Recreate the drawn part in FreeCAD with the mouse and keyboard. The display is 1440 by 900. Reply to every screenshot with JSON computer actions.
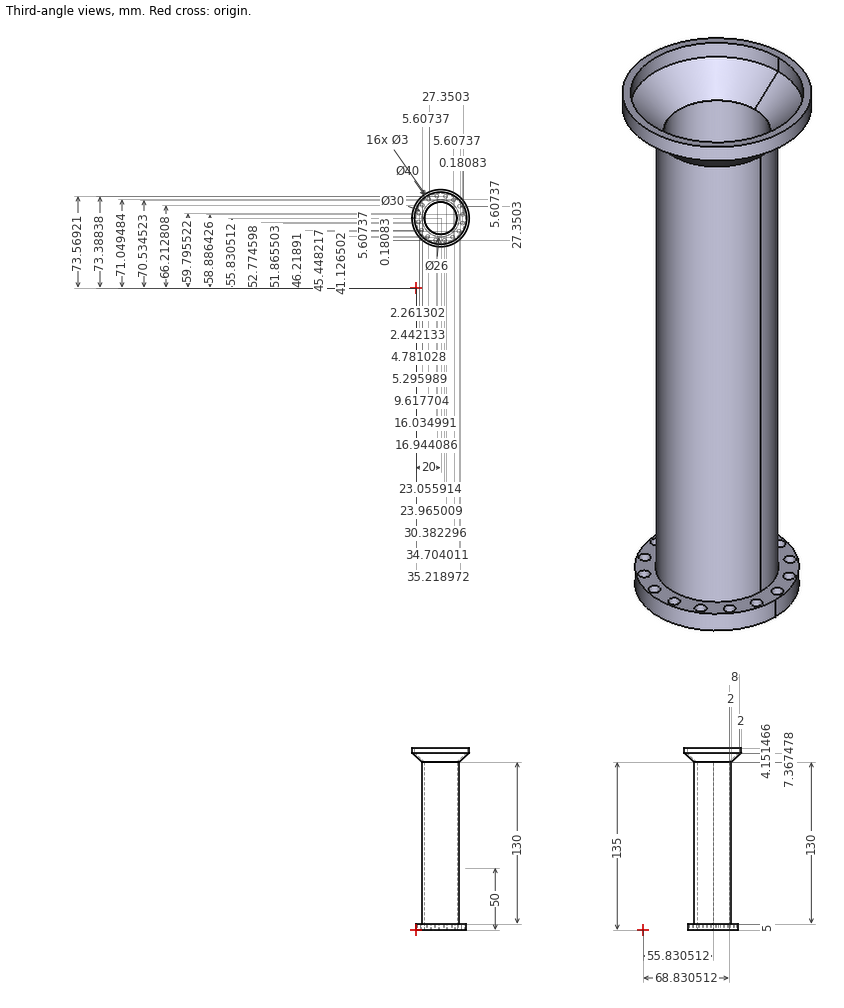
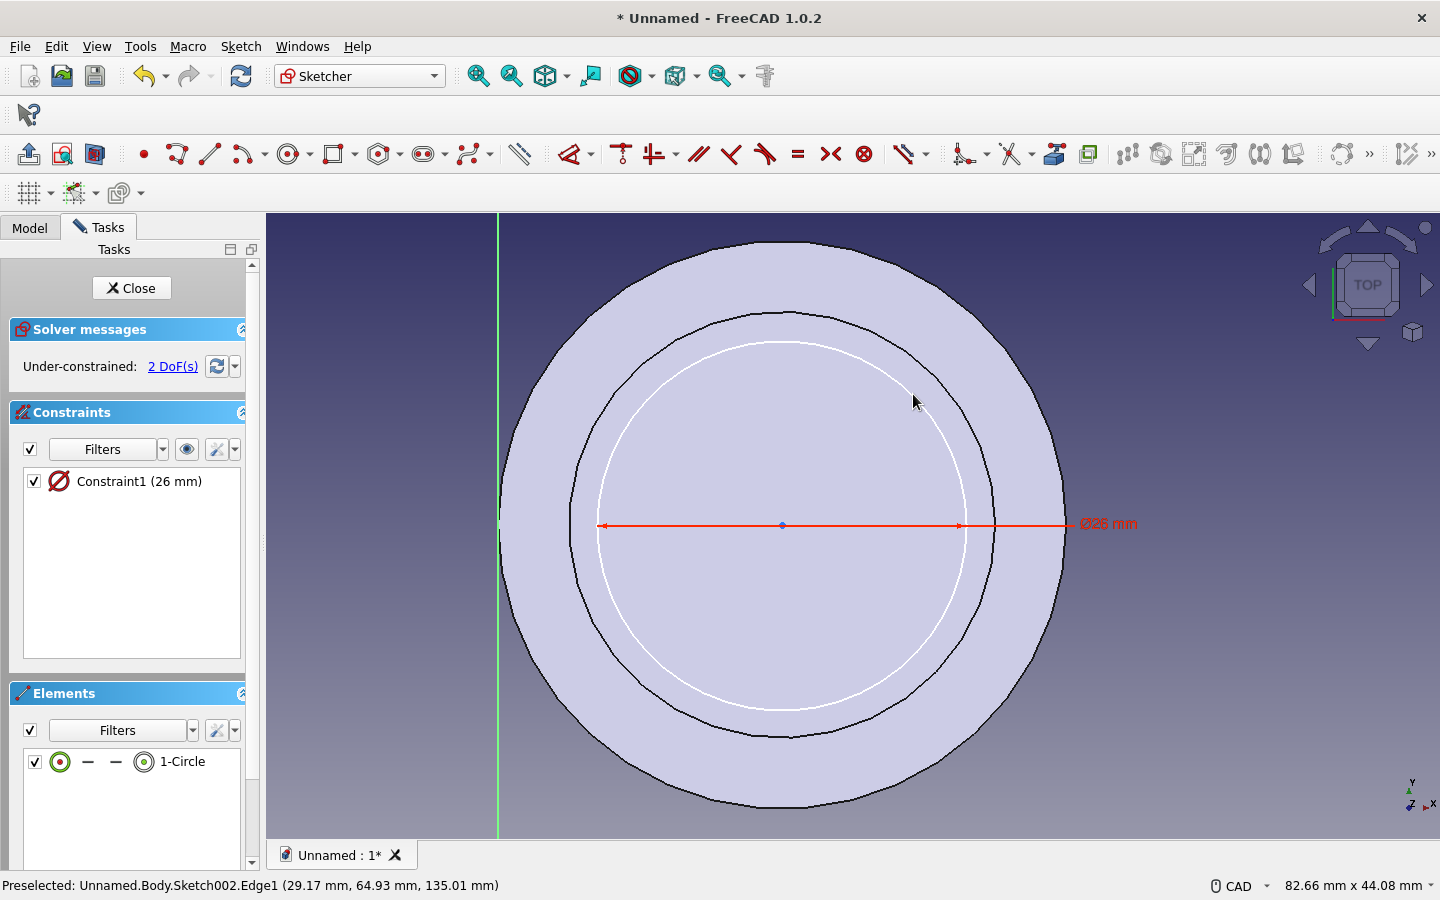
{"action": "key", "text": "d"}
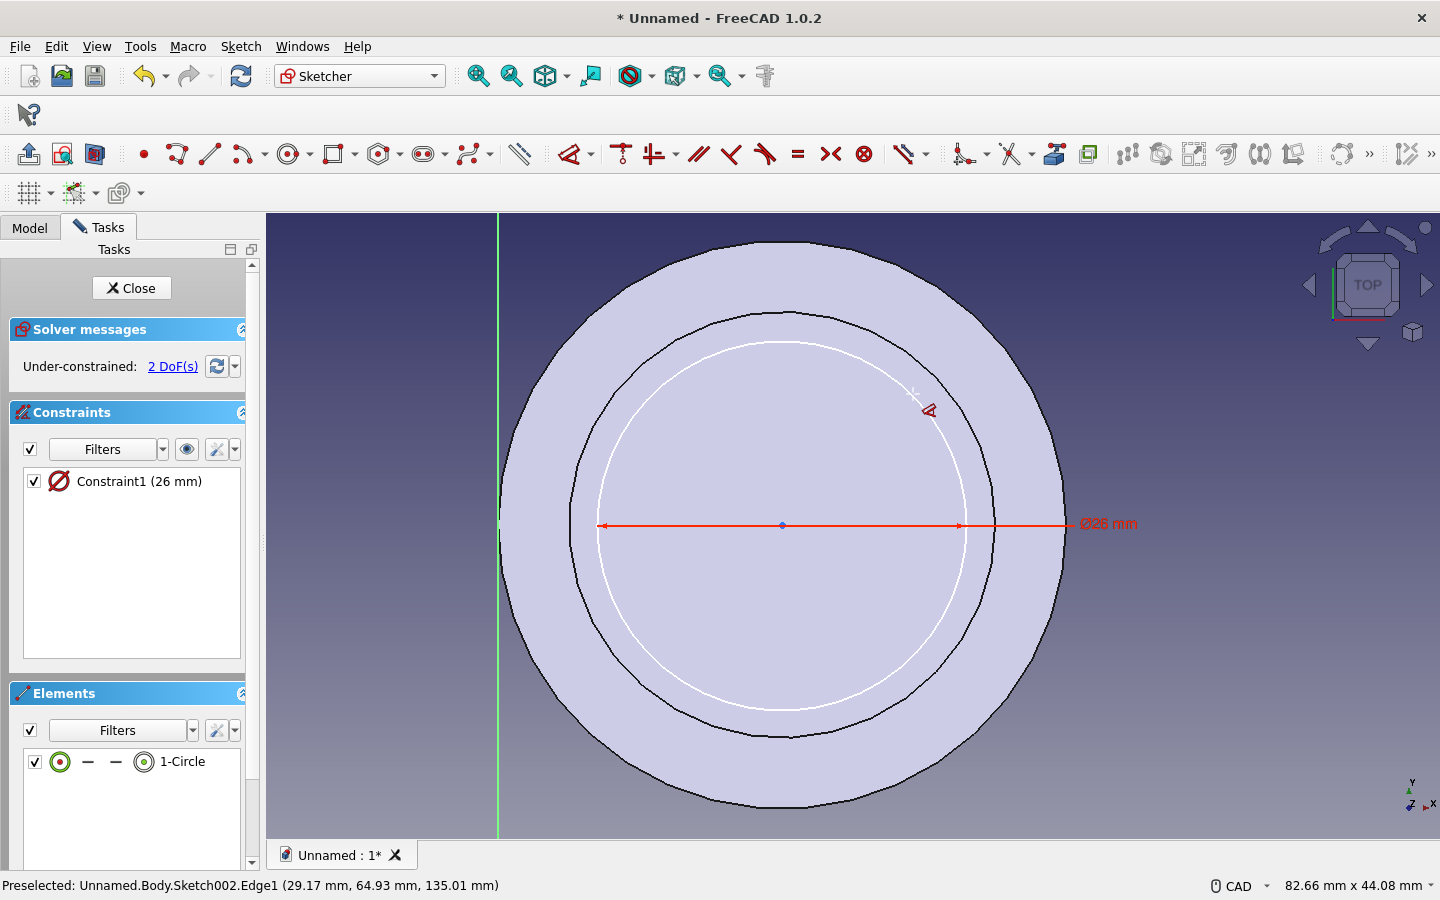
{"action": "left_click", "coordinate": [782, 526]}
{"action": "left_click", "coordinate": [640, 492]}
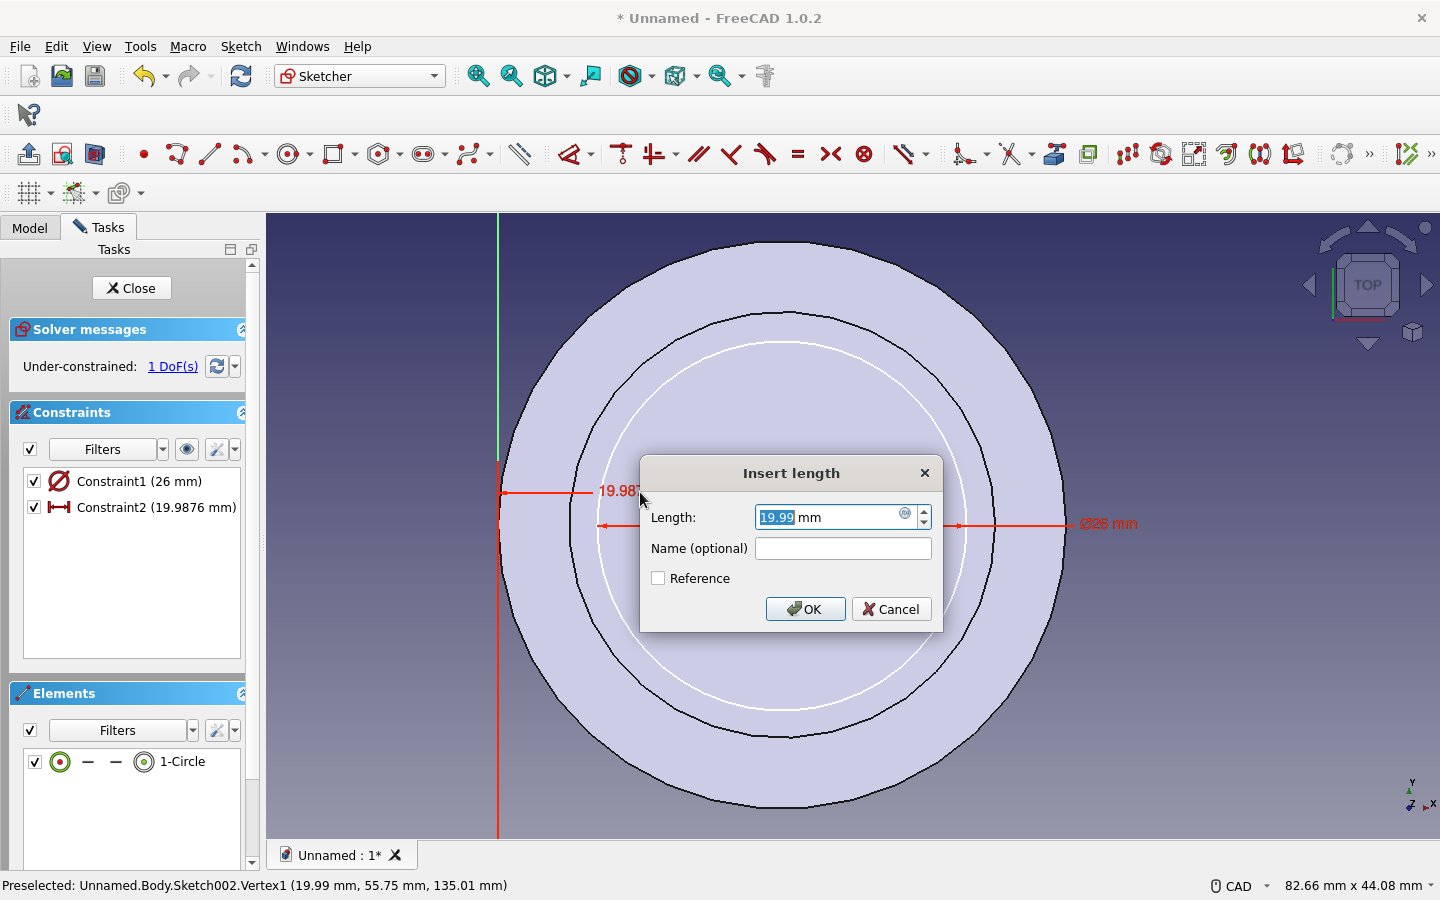
{"action": "type", "text": "20"}
{"action": "key", "text": "Return"}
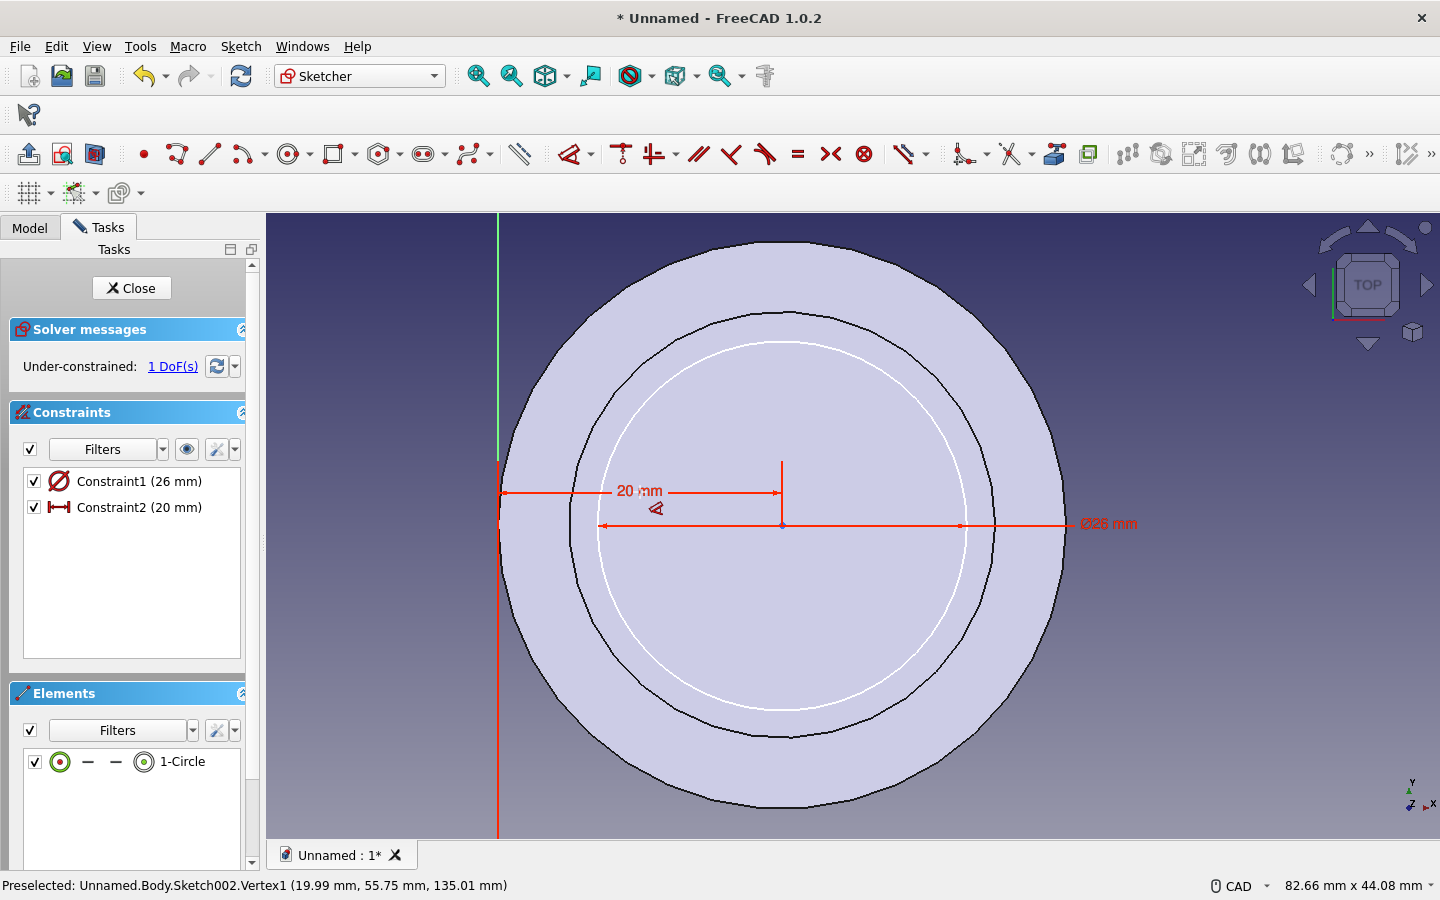
{"action": "left_click", "coordinate": [782, 526]}
{"action": "left_click", "coordinate": [464, 669]}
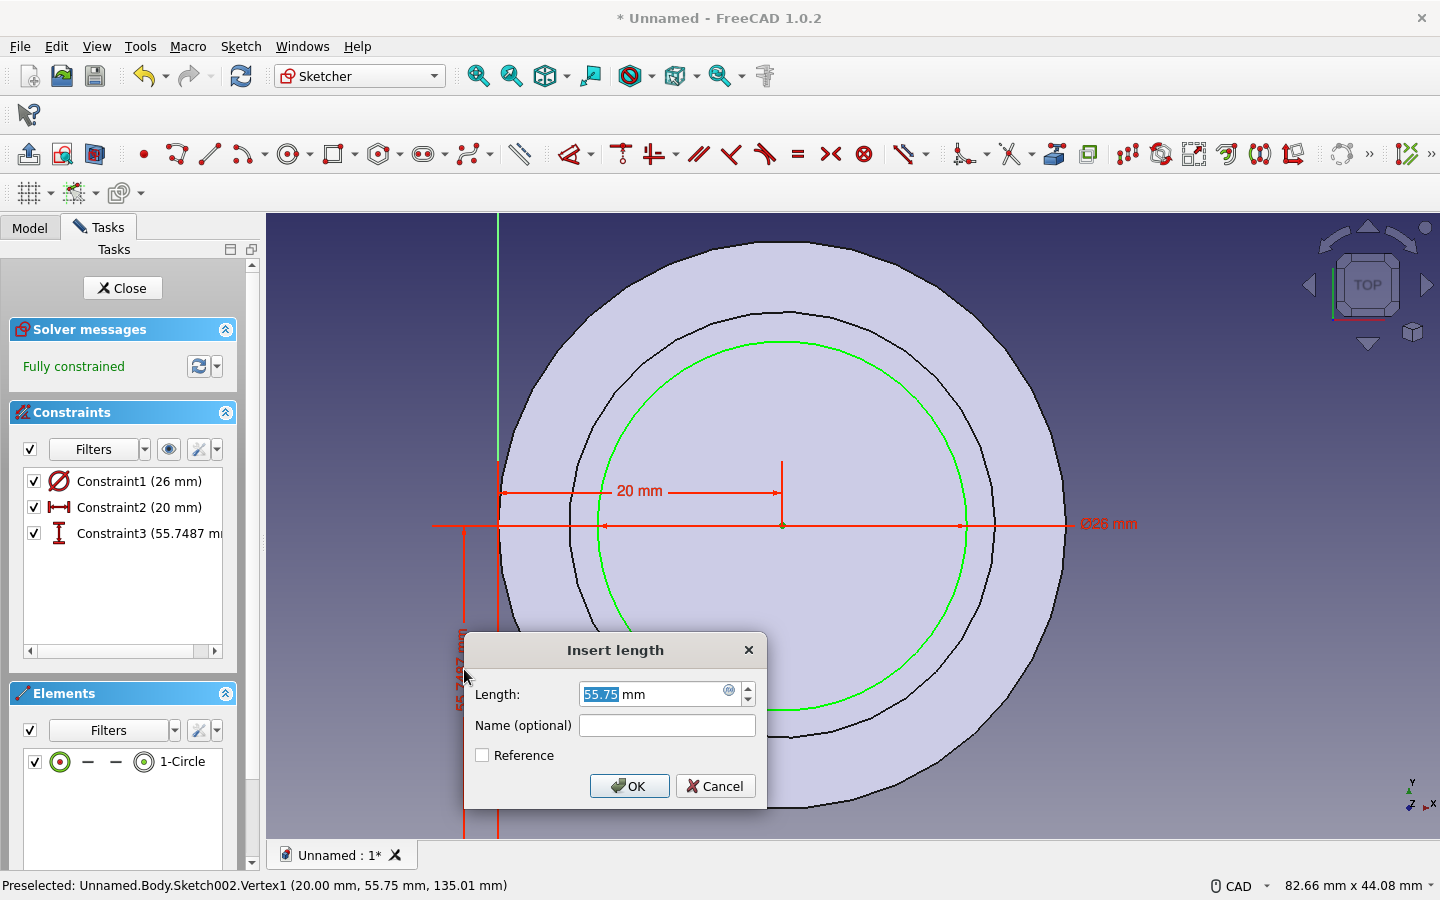
{"action": "type", "text": "55.830512"}
{"action": "key", "text": "Return"}
{"action": "key", "text": "Escape"}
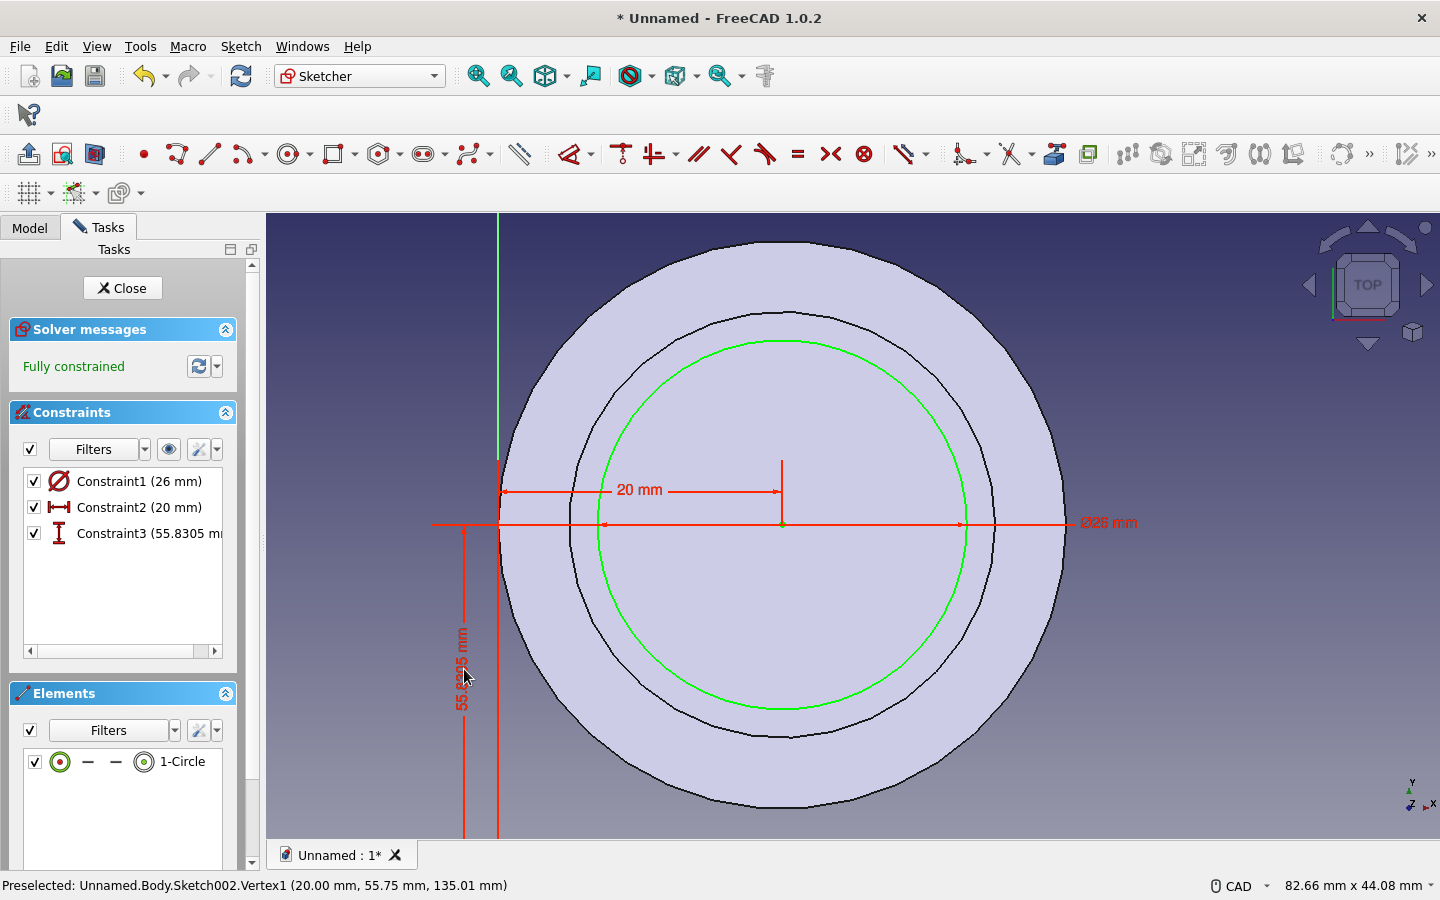
{"action": "left_click", "coordinate": [123, 288]}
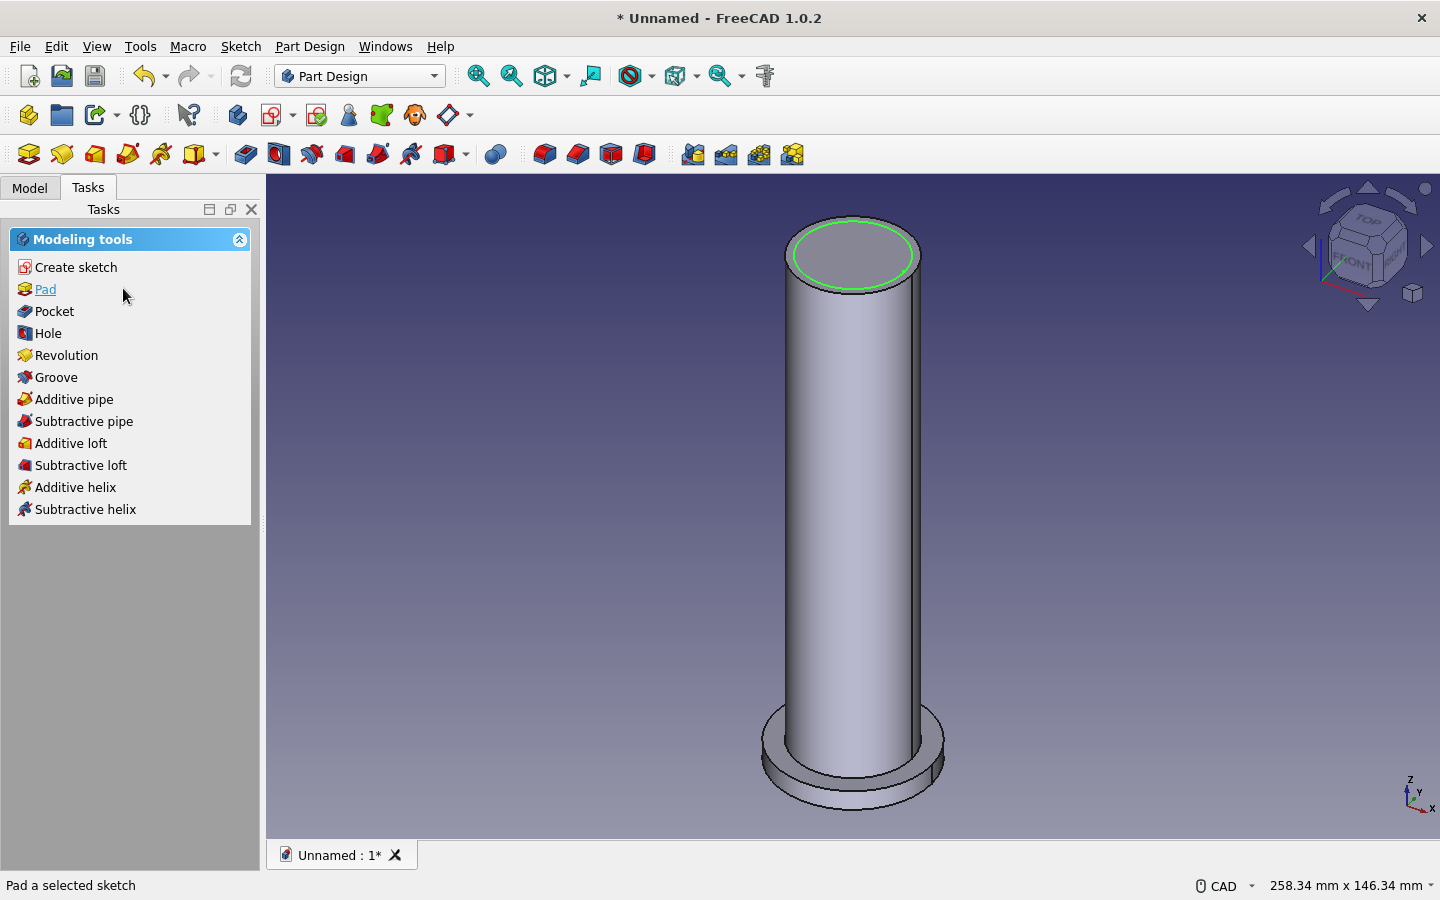
{"action": "left_click", "coordinate": [246, 154]}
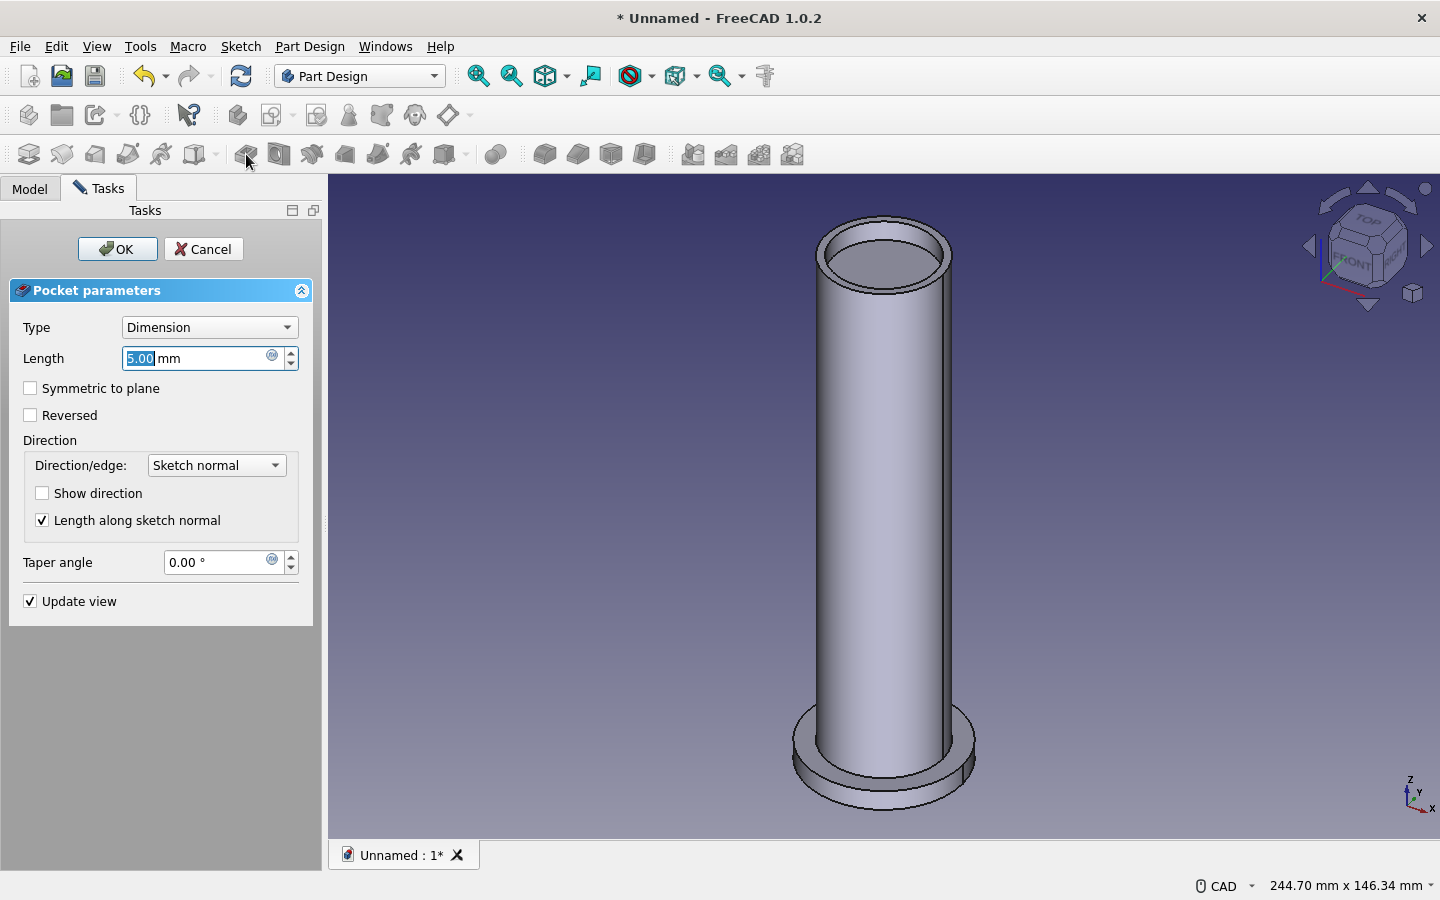
{"action": "left_click", "coordinate": [210, 328]}